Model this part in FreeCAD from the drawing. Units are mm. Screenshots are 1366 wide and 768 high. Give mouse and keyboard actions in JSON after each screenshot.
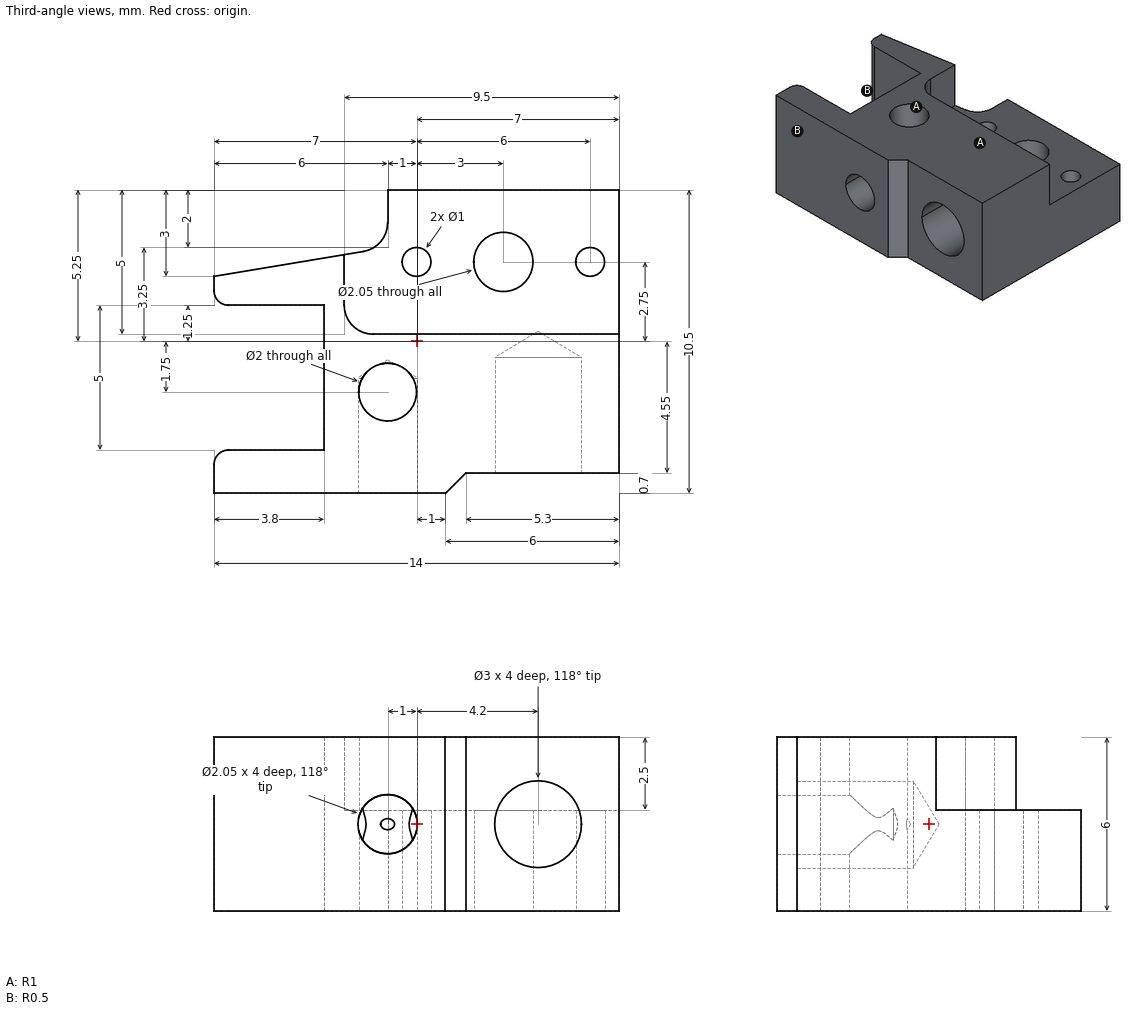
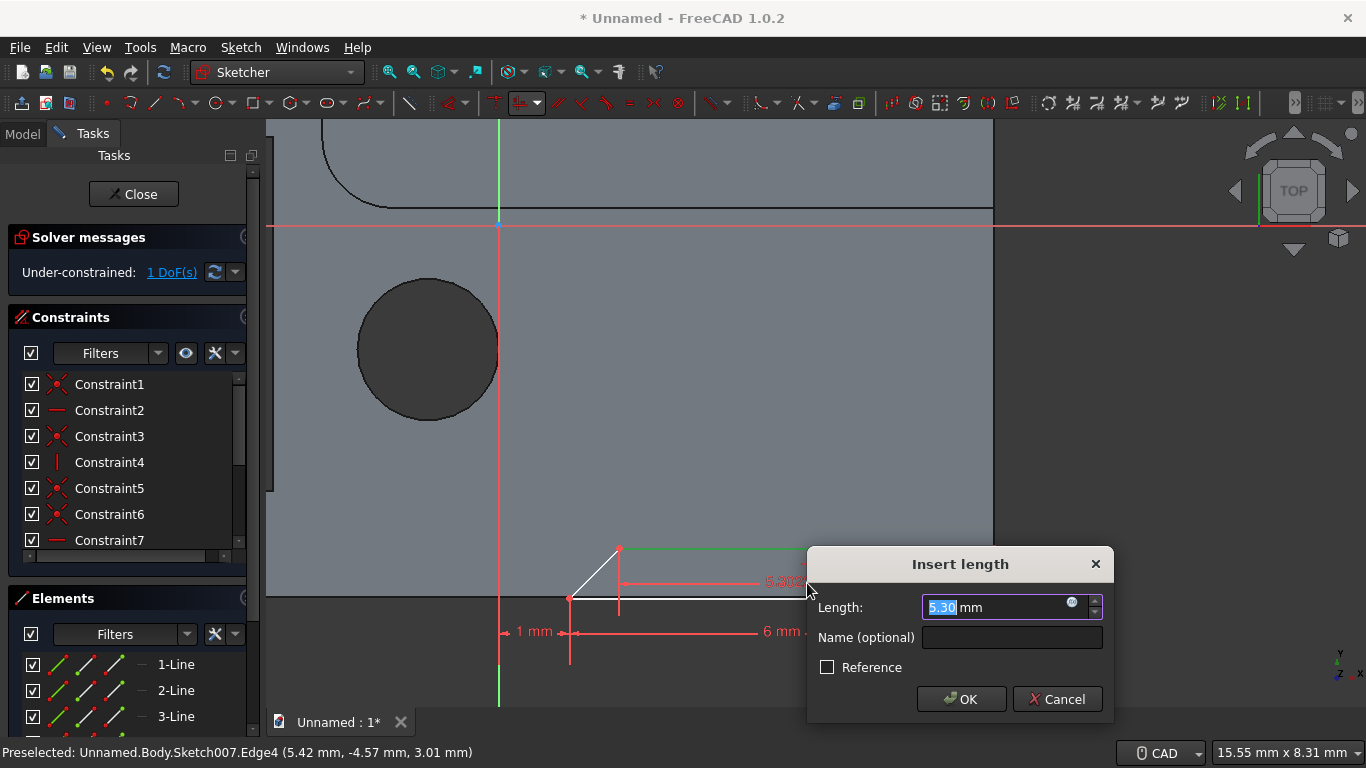
{"action": "type", "text": "5.3"}
{"action": "key", "text": "Return"}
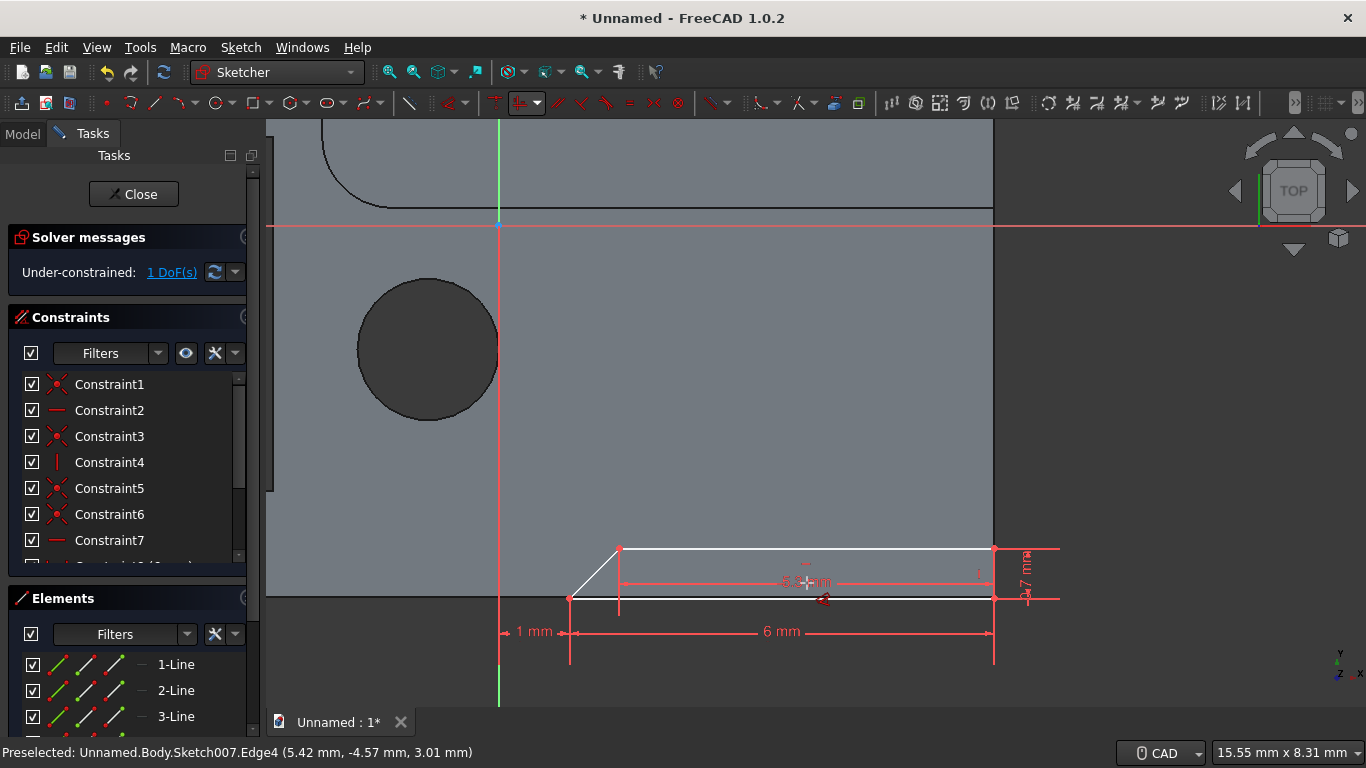
{"action": "left_click", "coordinate": [619, 549]}
{"action": "left_click", "coordinate": [465, 387]}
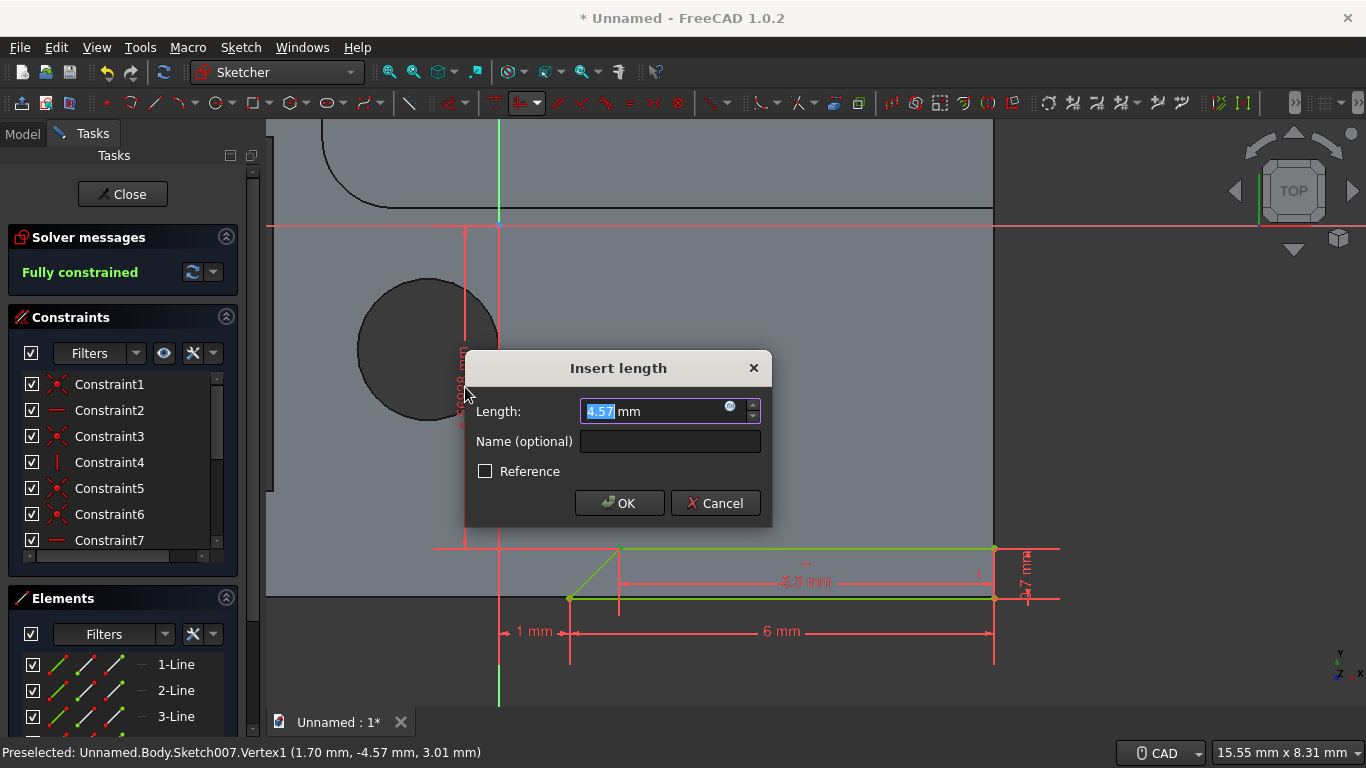
{"action": "type", "text": "4.55"}
{"action": "key", "text": "Return"}
{"action": "key", "text": "Escape"}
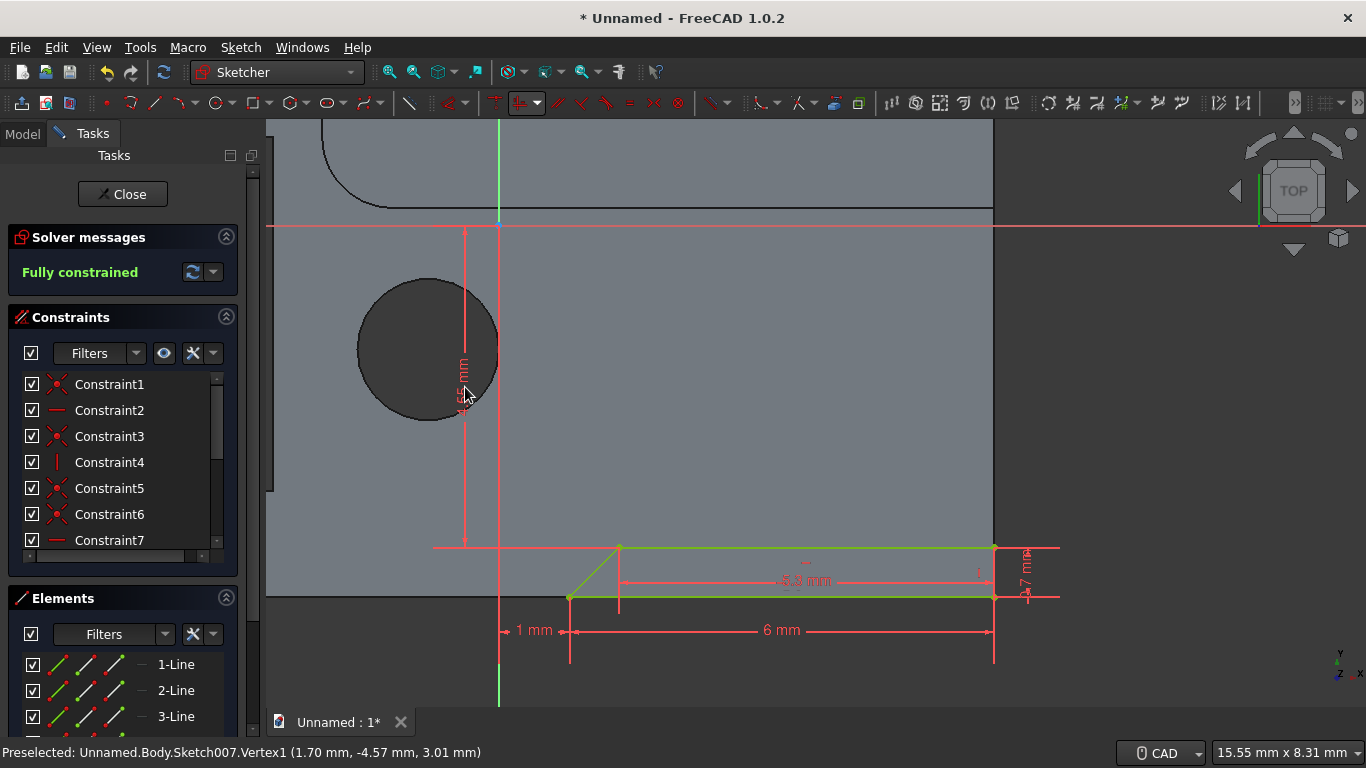
{"action": "left_click", "coordinate": [123, 194]}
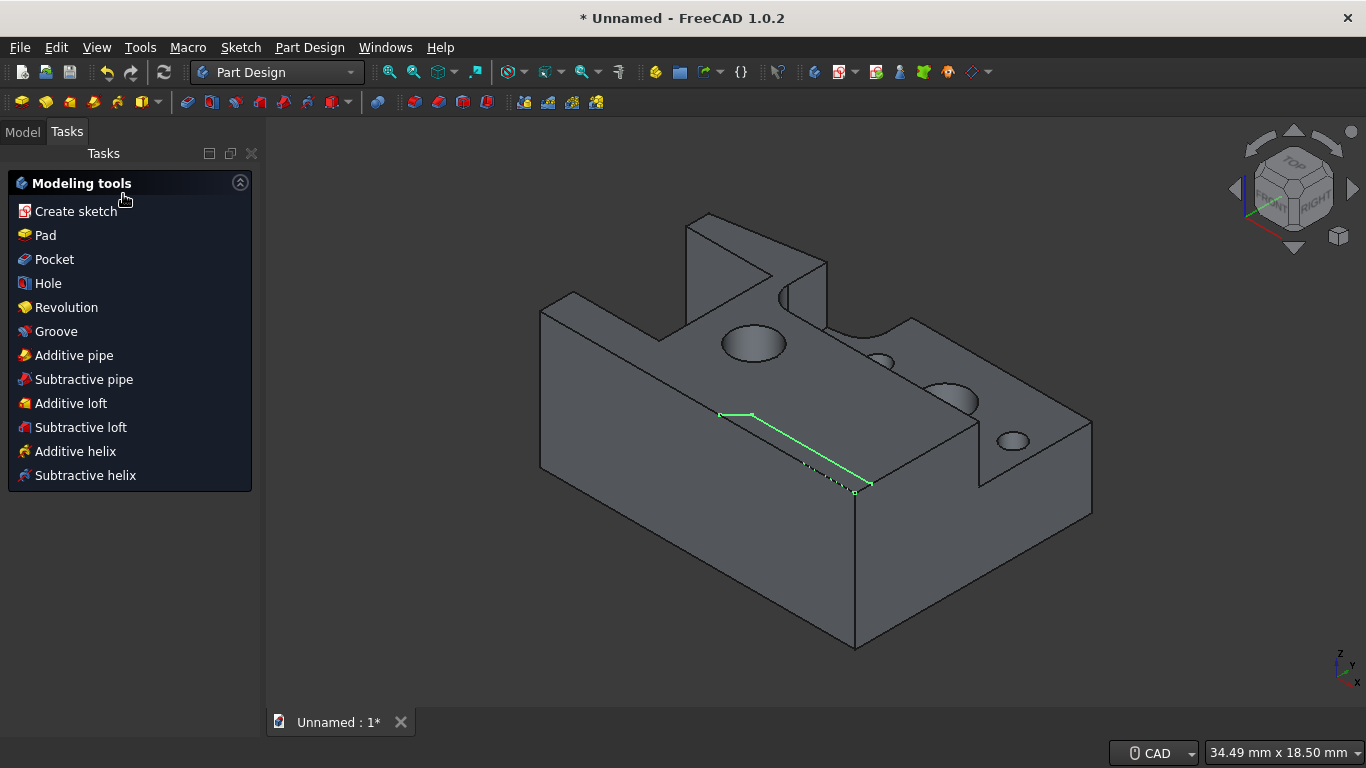
{"action": "left_click", "coordinate": [188, 102]}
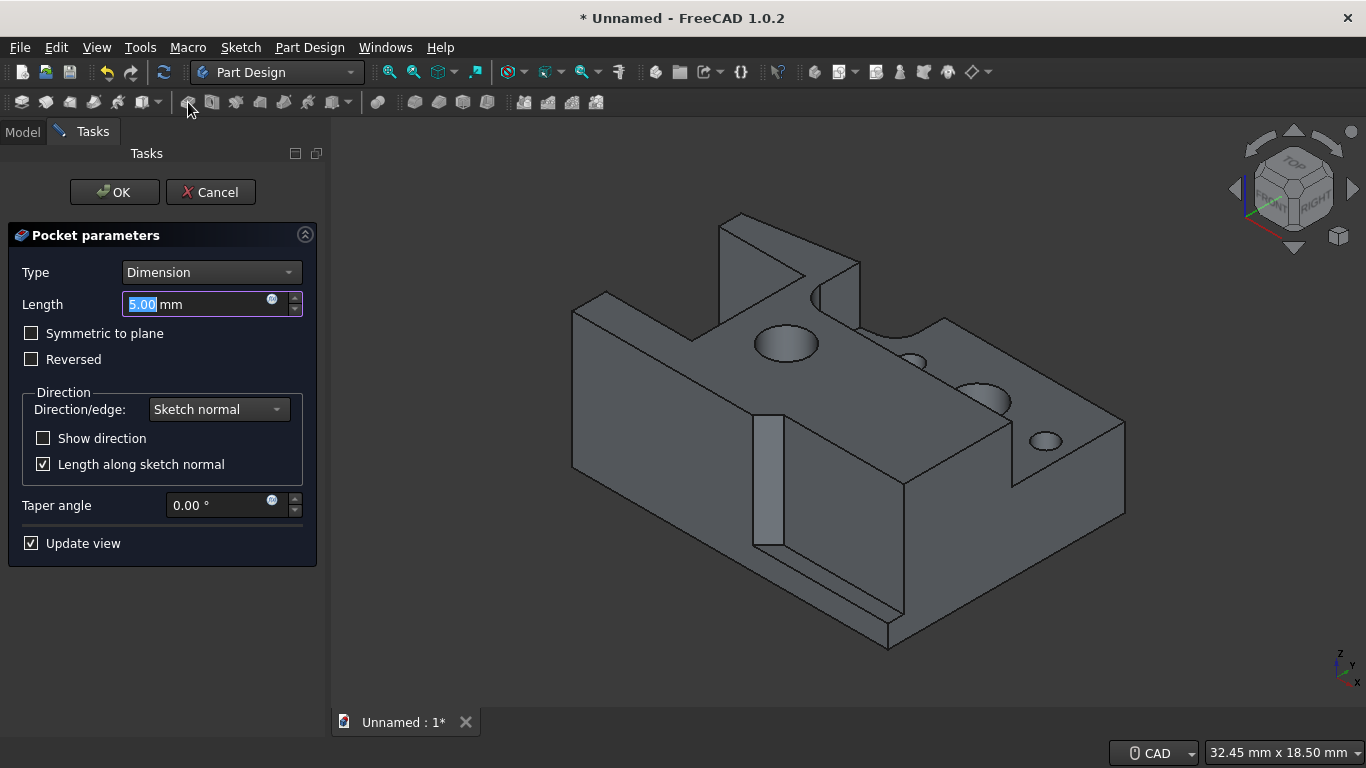
{"action": "left_click", "coordinate": [212, 272]}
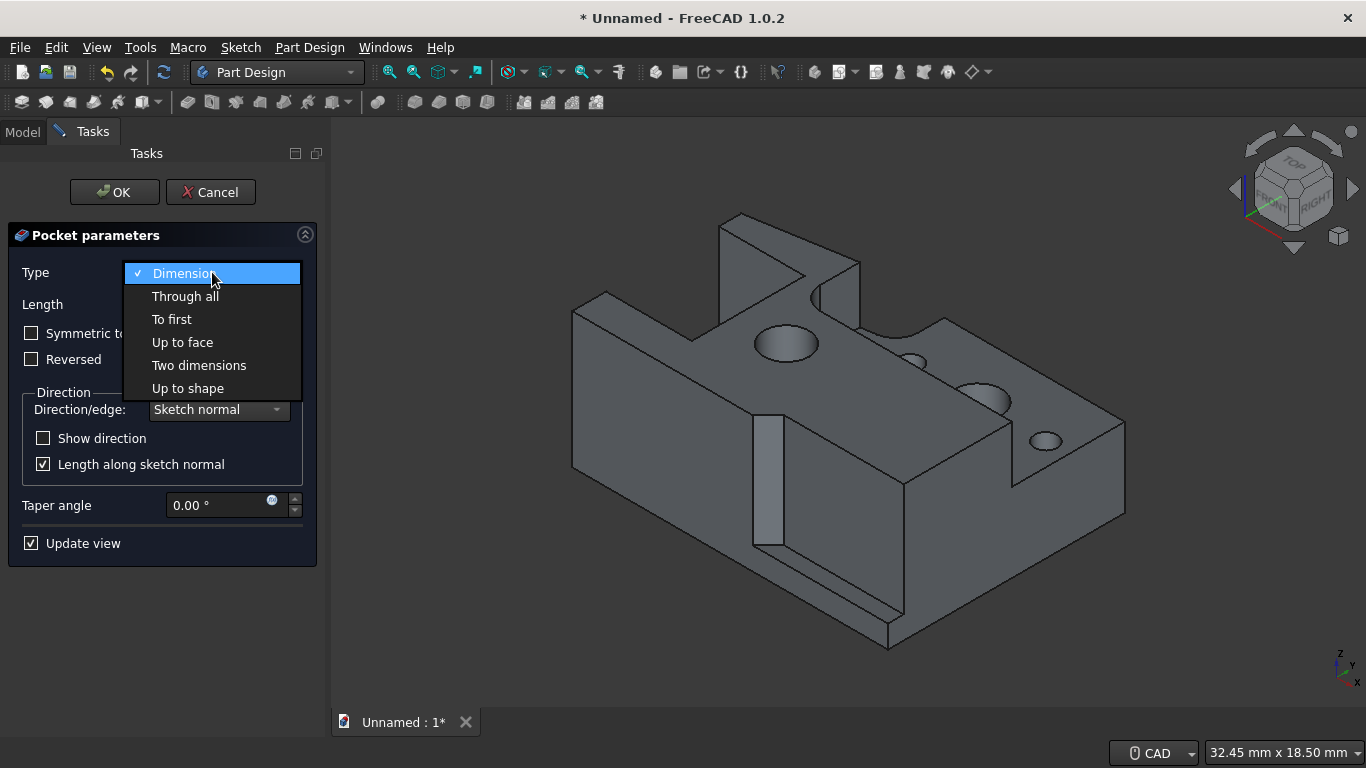
{"action": "left_click", "coordinate": [212, 296]}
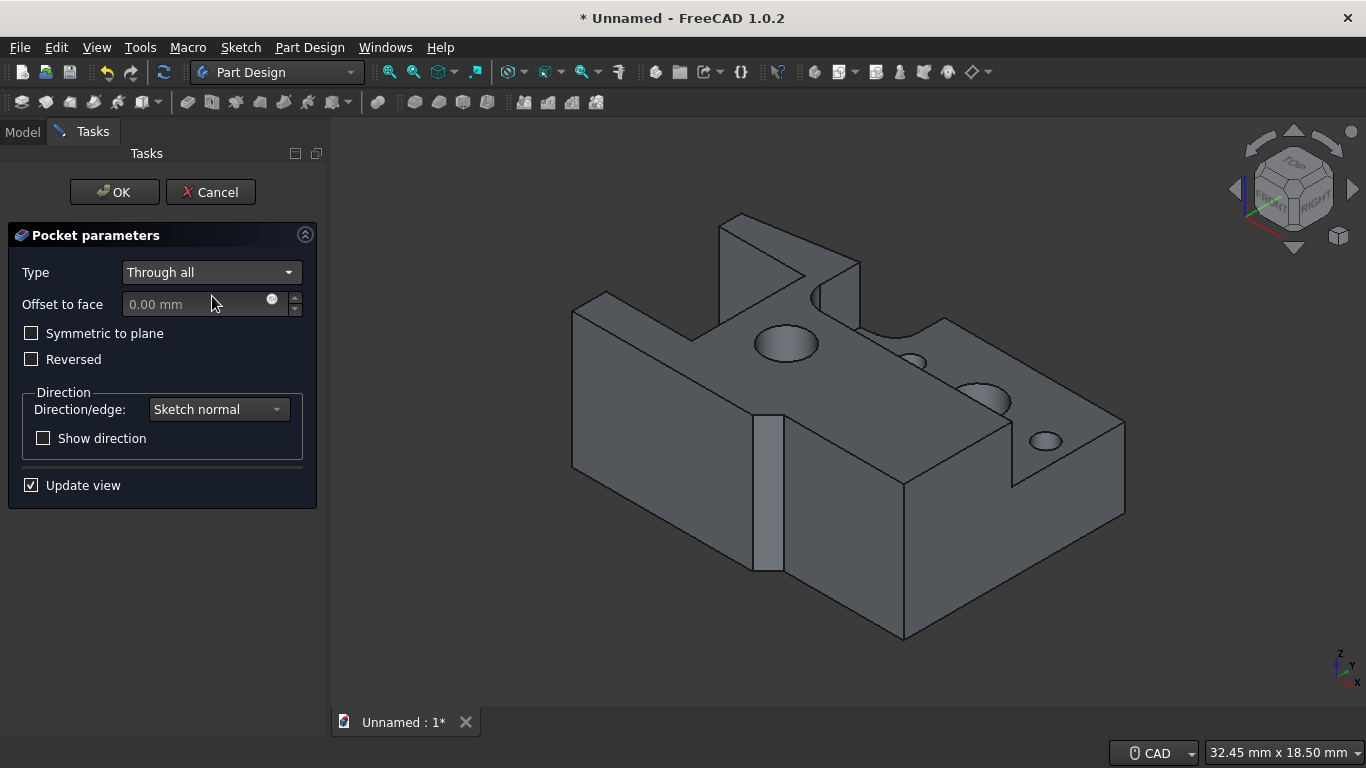
{"action": "left_click", "coordinate": [115, 192]}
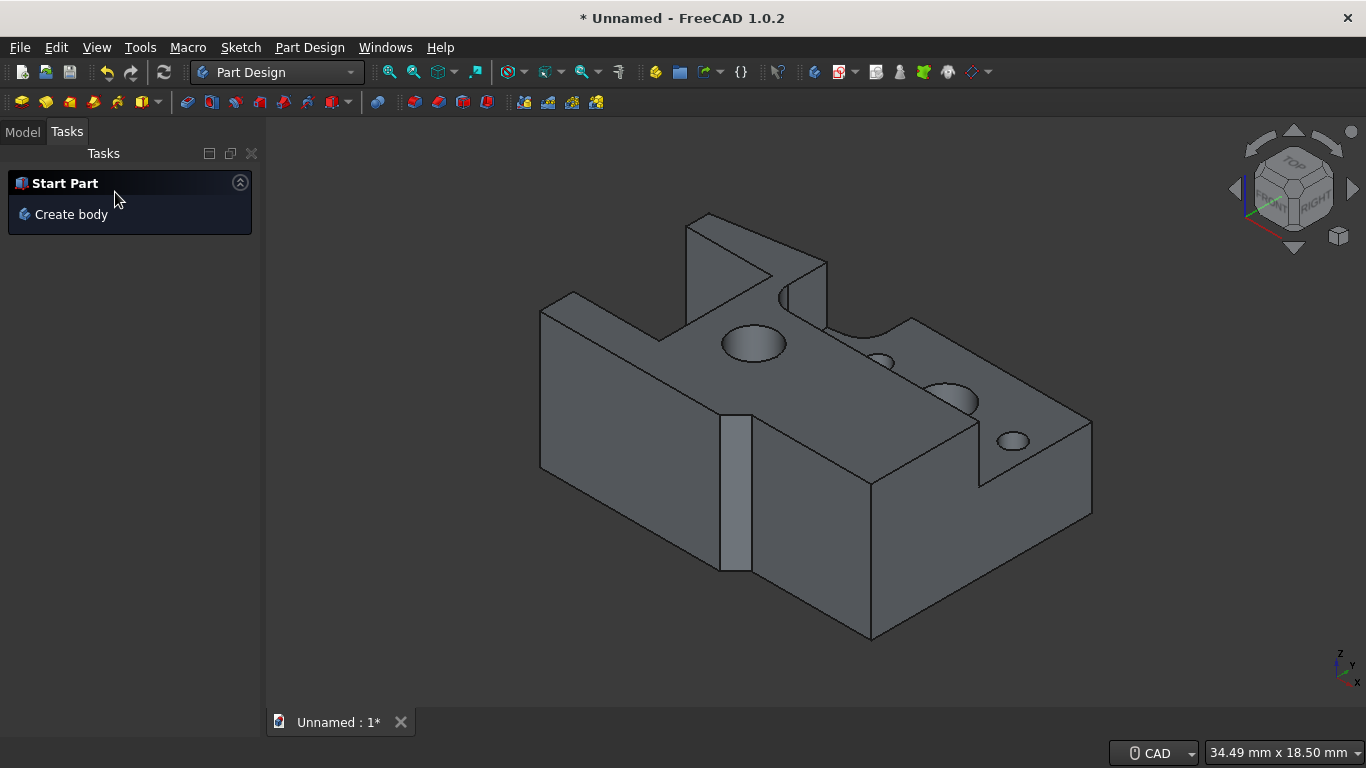
{"action": "left_click", "coordinate": [811, 527]}